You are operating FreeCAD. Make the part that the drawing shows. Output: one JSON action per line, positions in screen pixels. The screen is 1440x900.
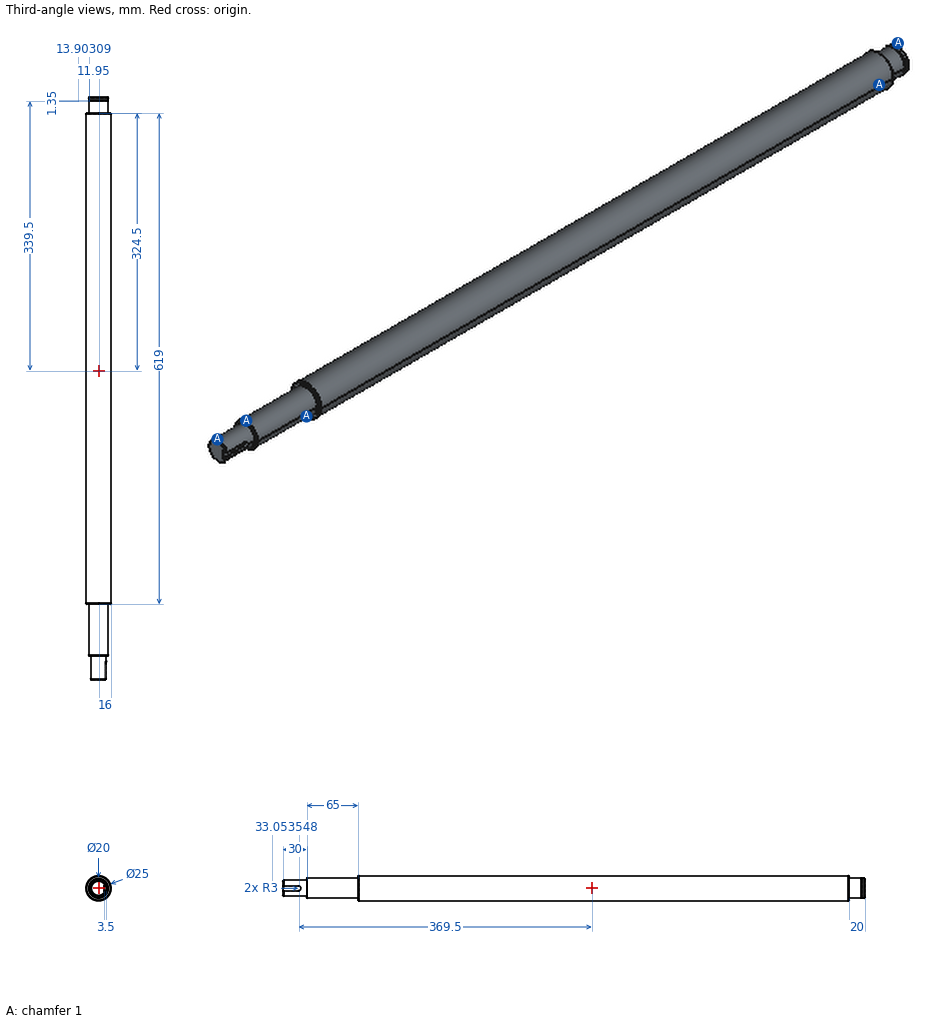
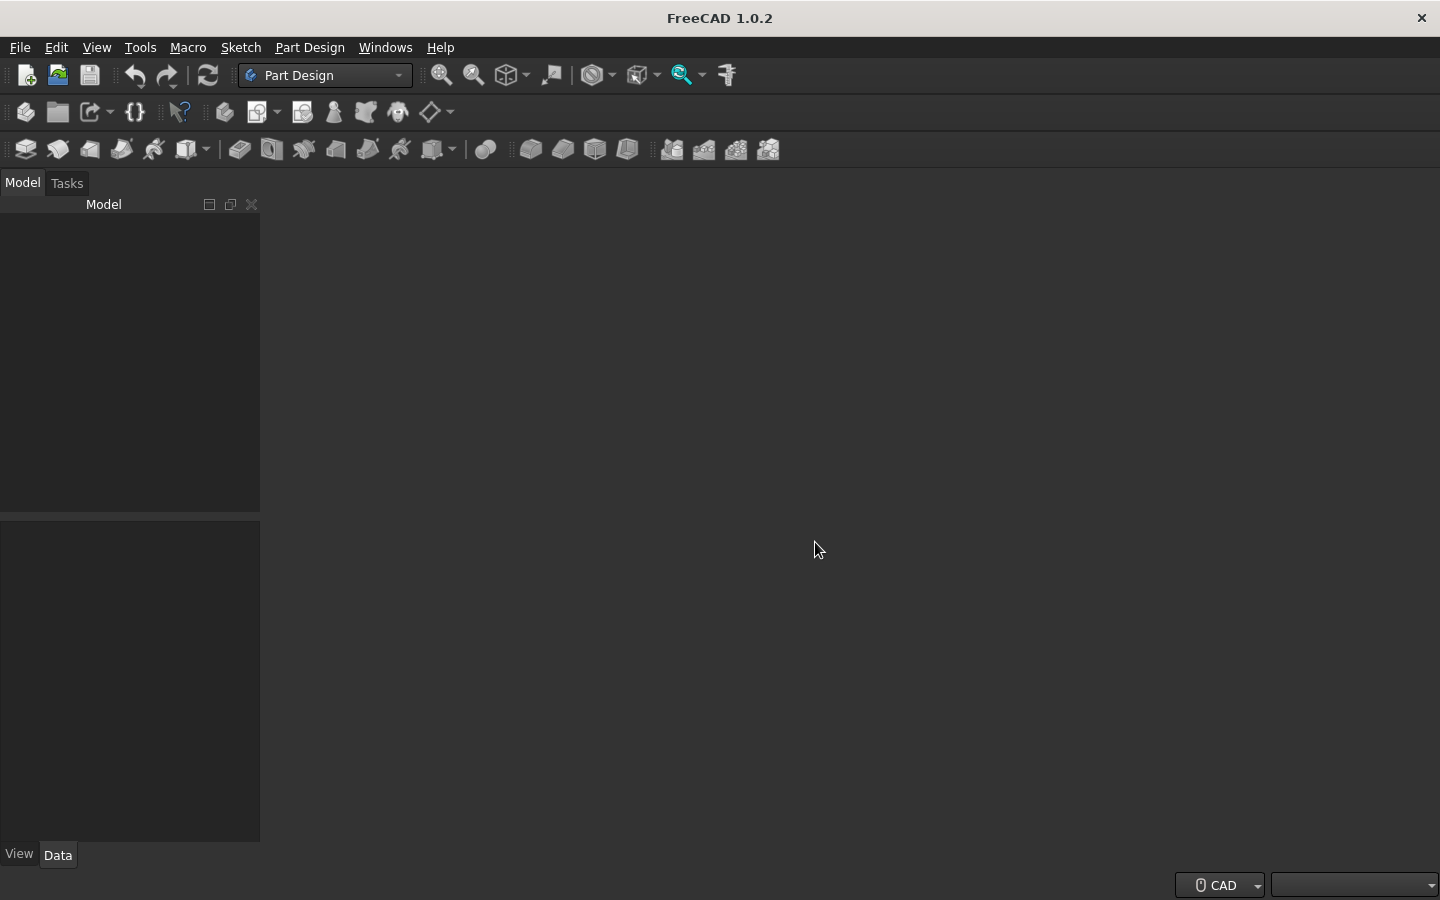
{"action": "left_click", "coordinate": [26, 76]}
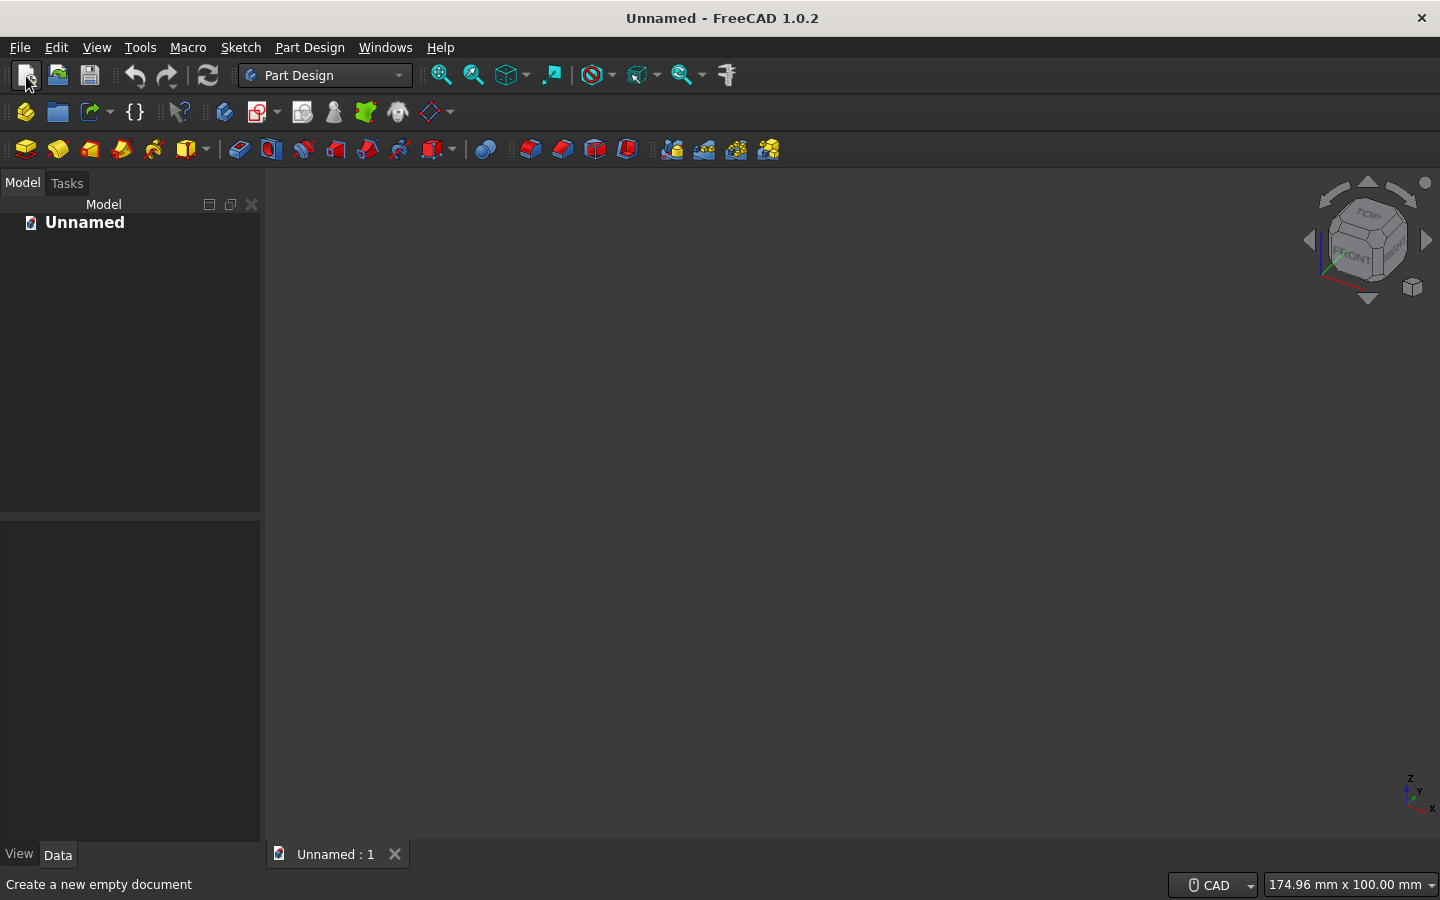
{"action": "left_click", "coordinate": [258, 112]}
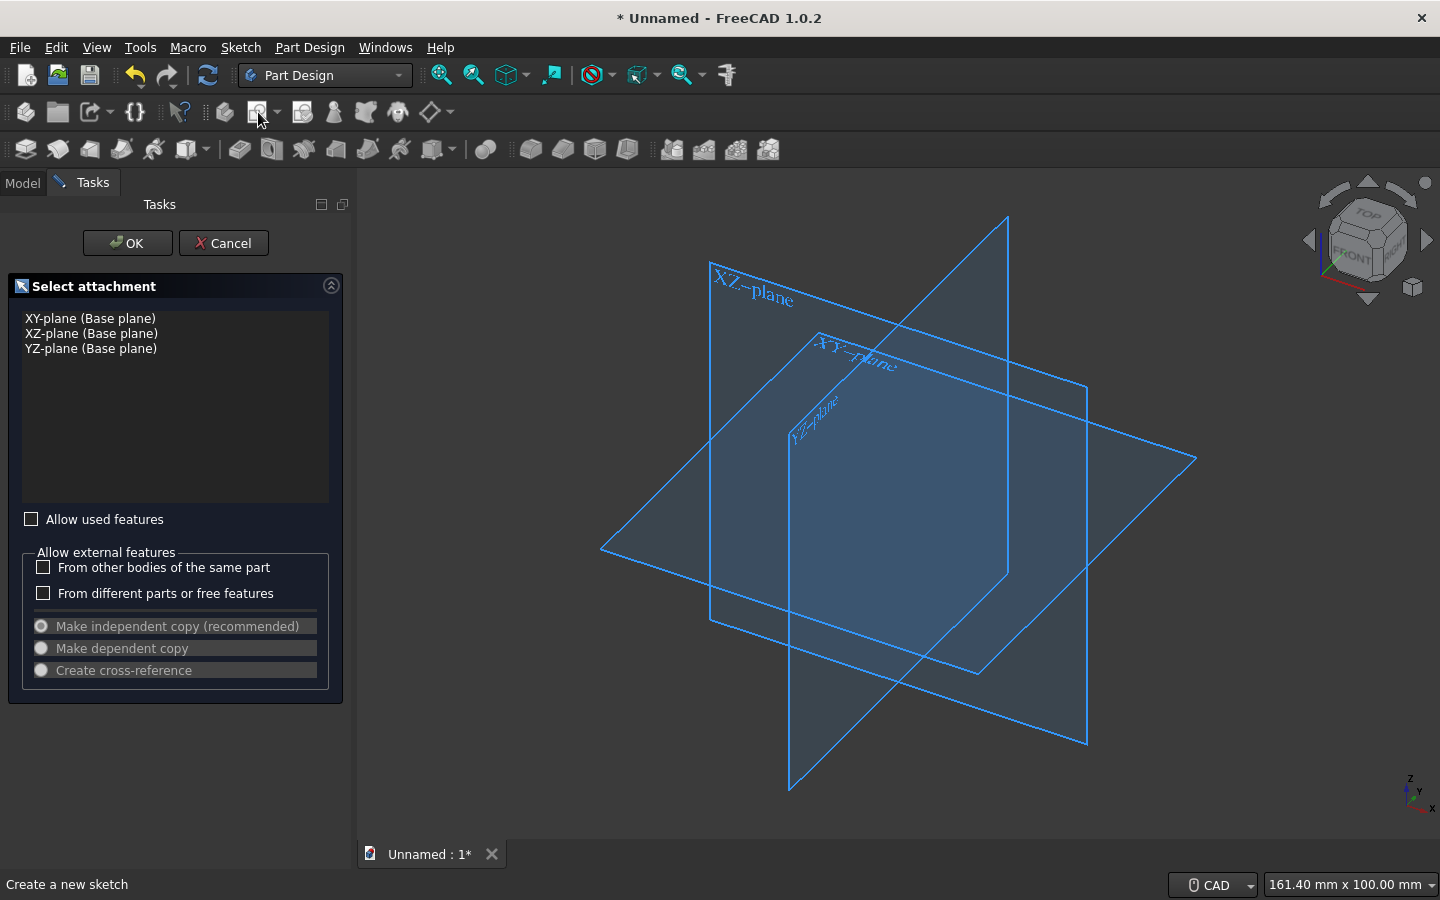
{"action": "left_click", "coordinate": [82, 318]}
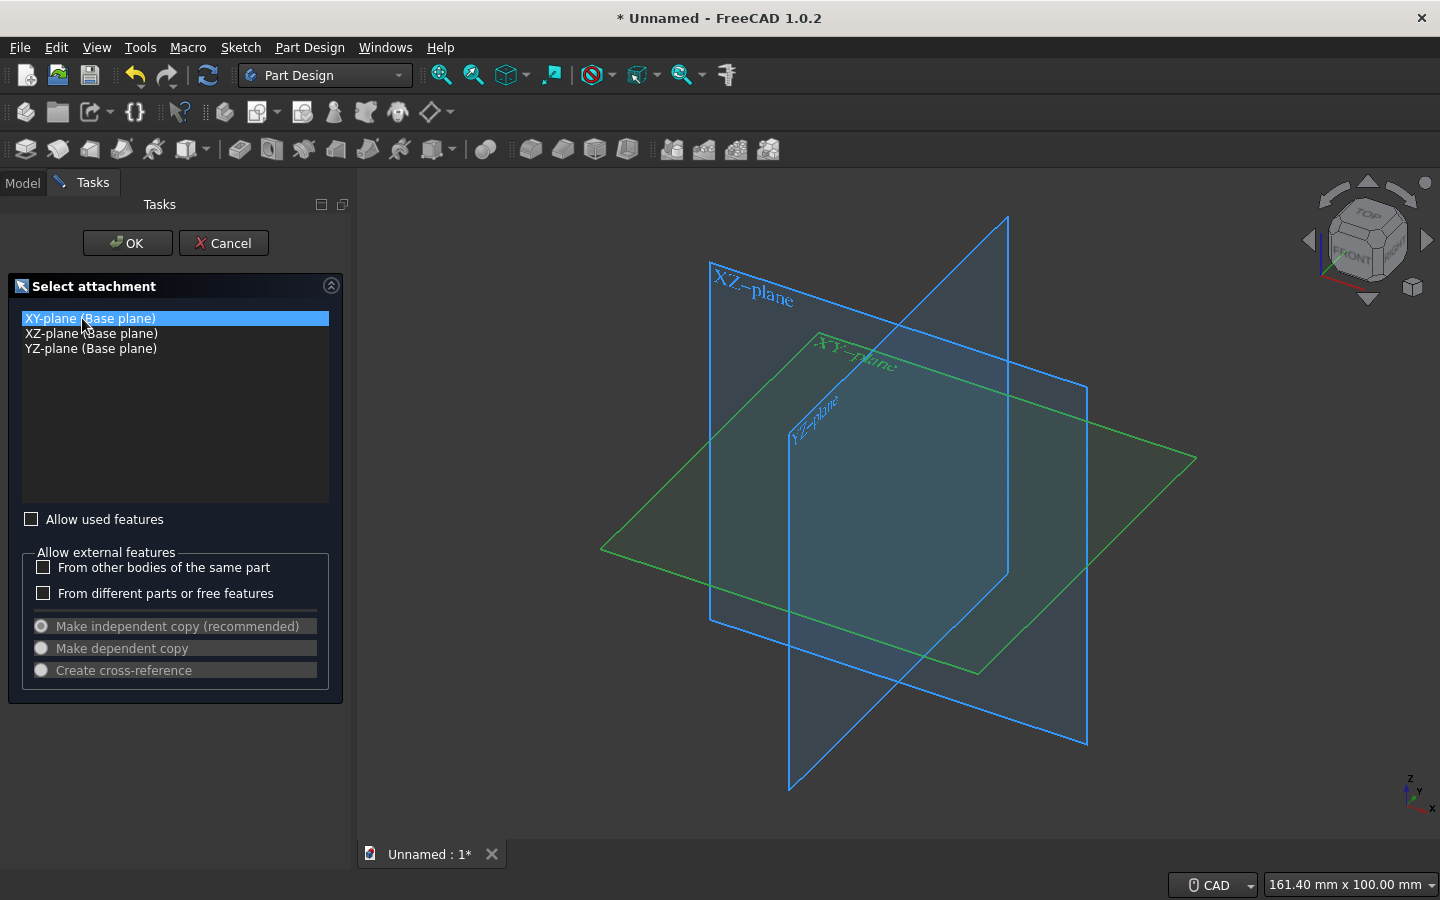
{"action": "left_click", "coordinate": [128, 243]}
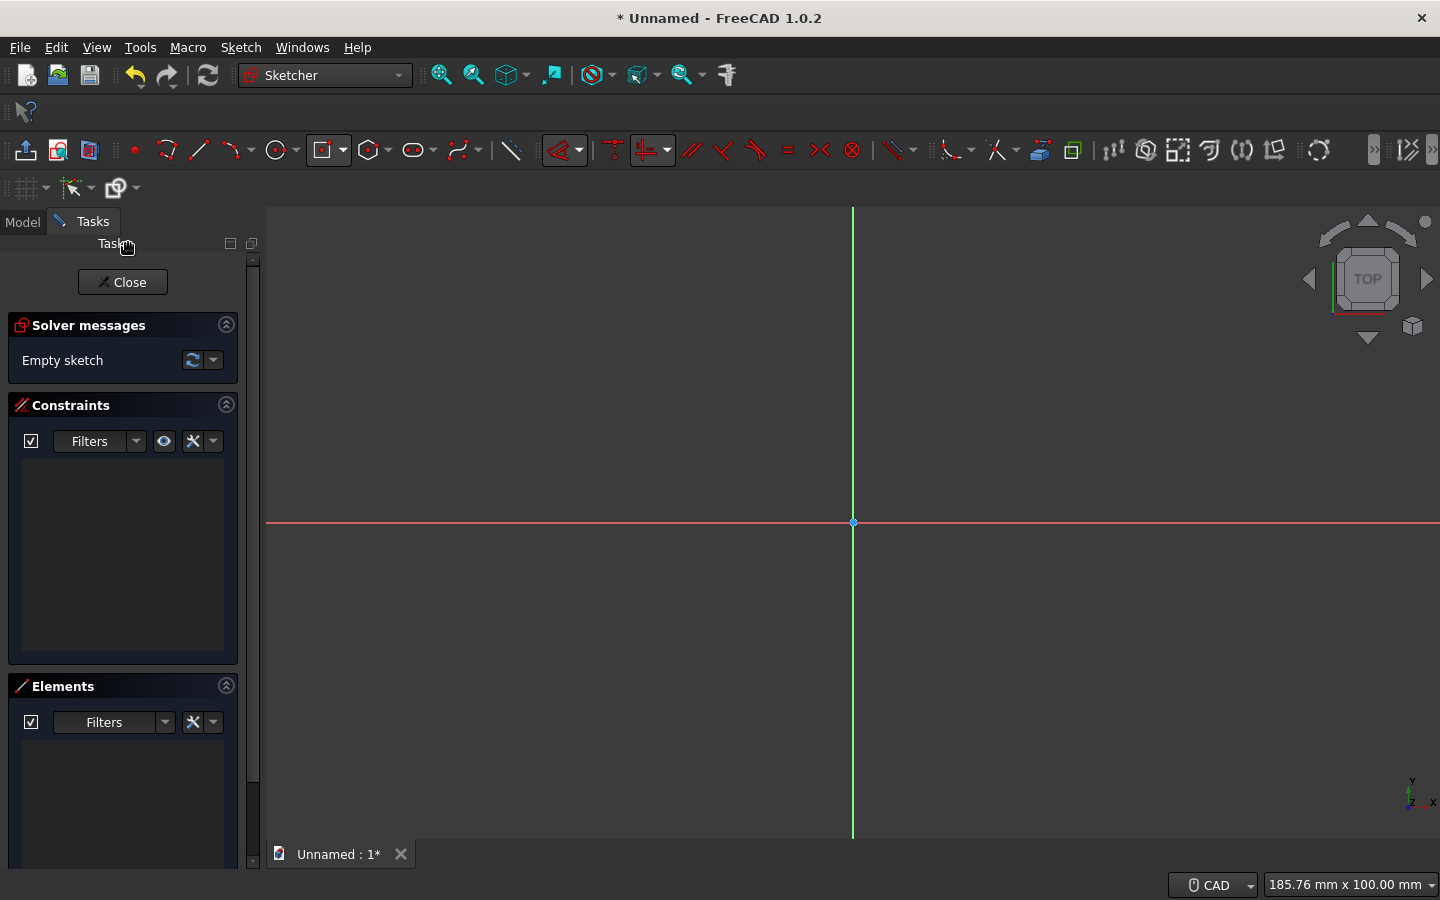
{"action": "scroll", "coordinate": [770, 535], "scroll_direction": "down", "scroll_amount": 11}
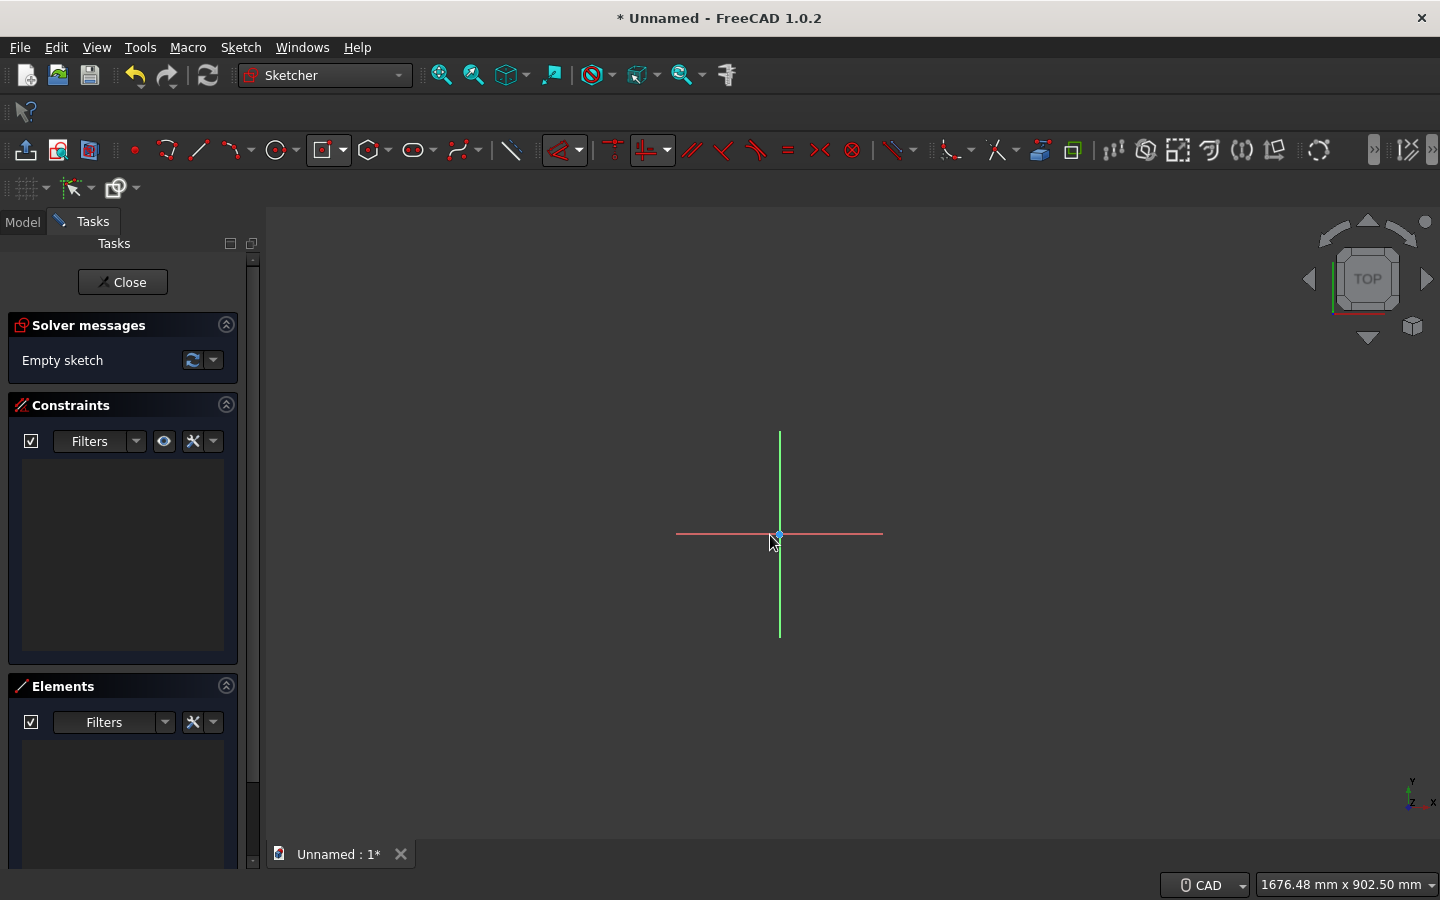
{"action": "left_click", "coordinate": [346, 150]}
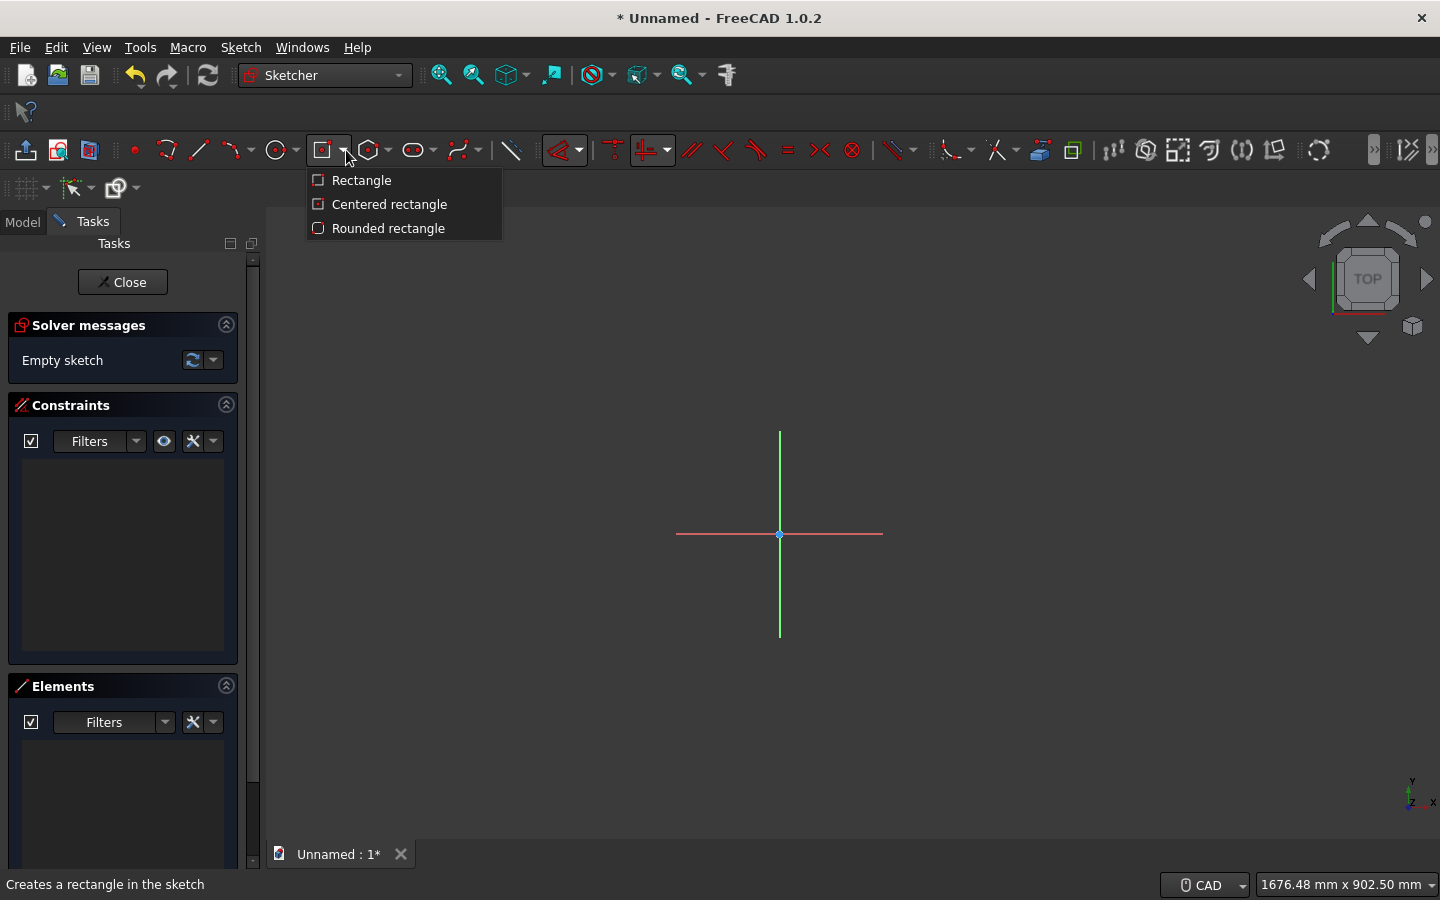
{"action": "left_click", "coordinate": [404, 180]}